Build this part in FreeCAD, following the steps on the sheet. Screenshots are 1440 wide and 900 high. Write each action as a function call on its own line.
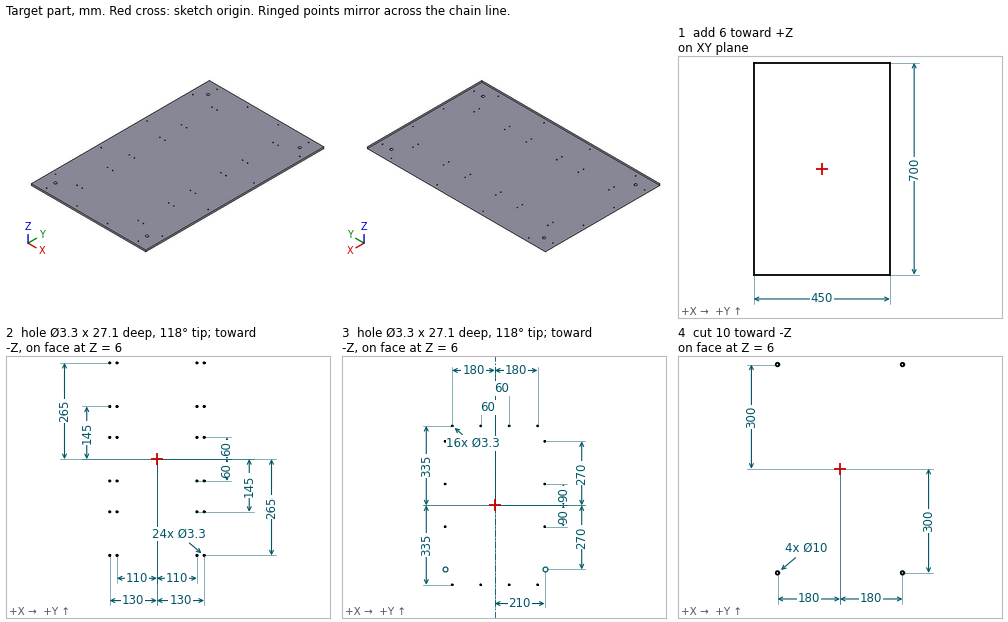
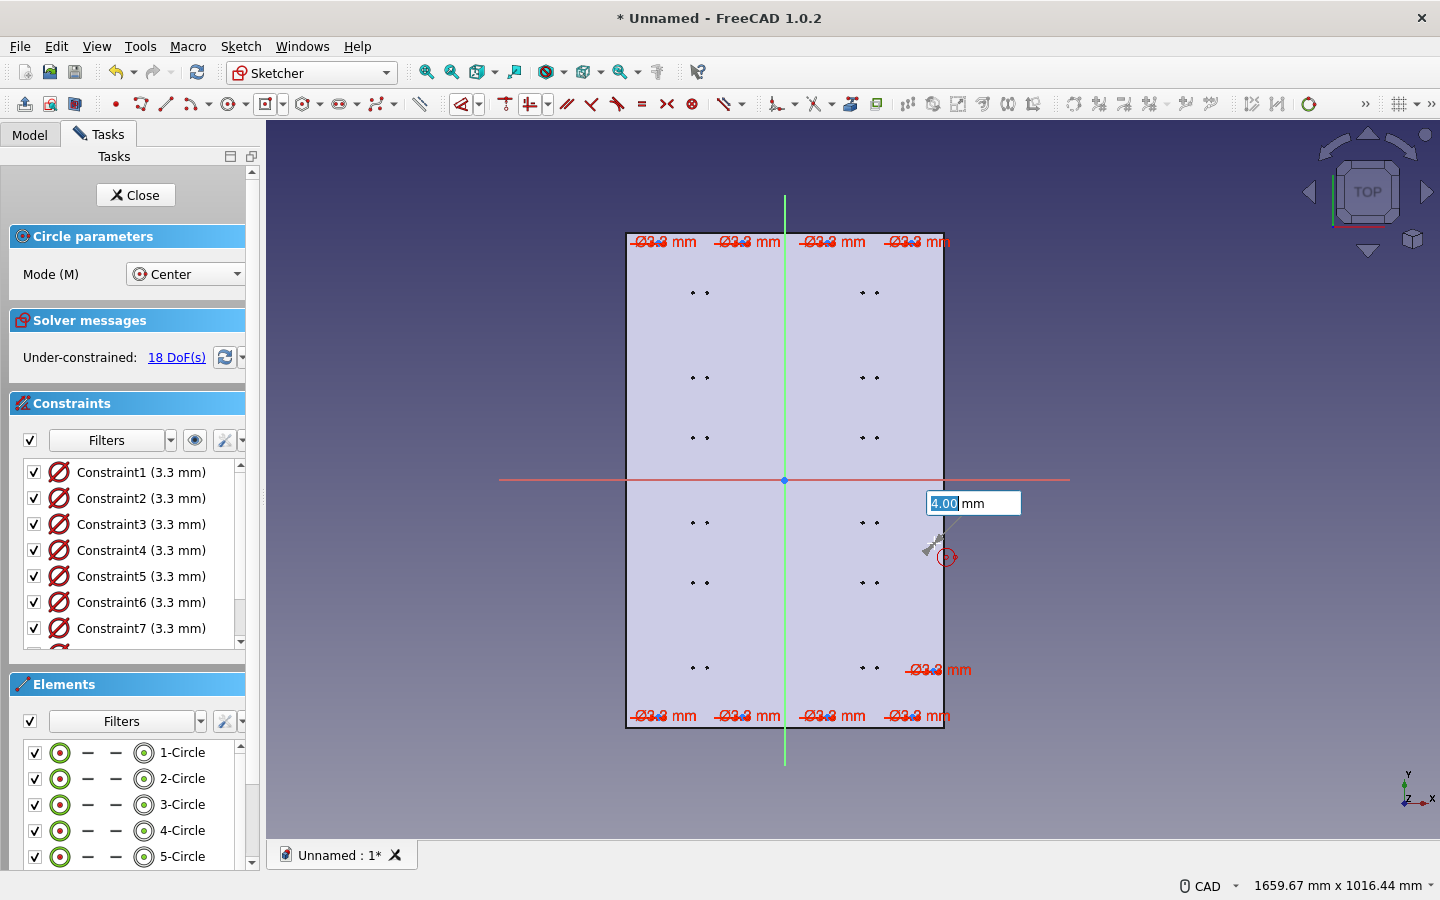
text(3.3)
key(Return)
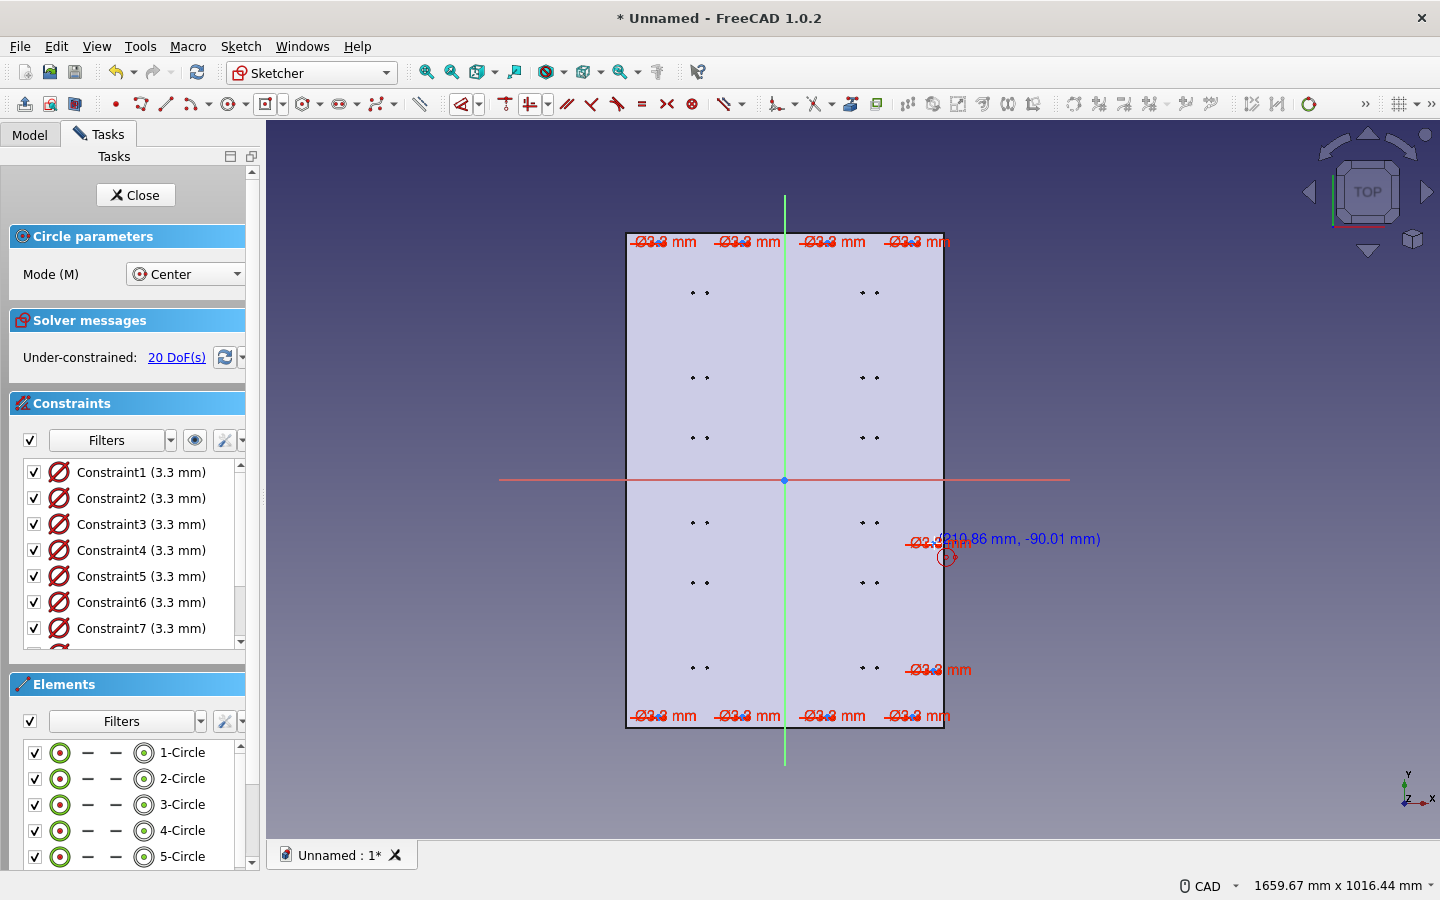
scroll(933, 417, up, 15)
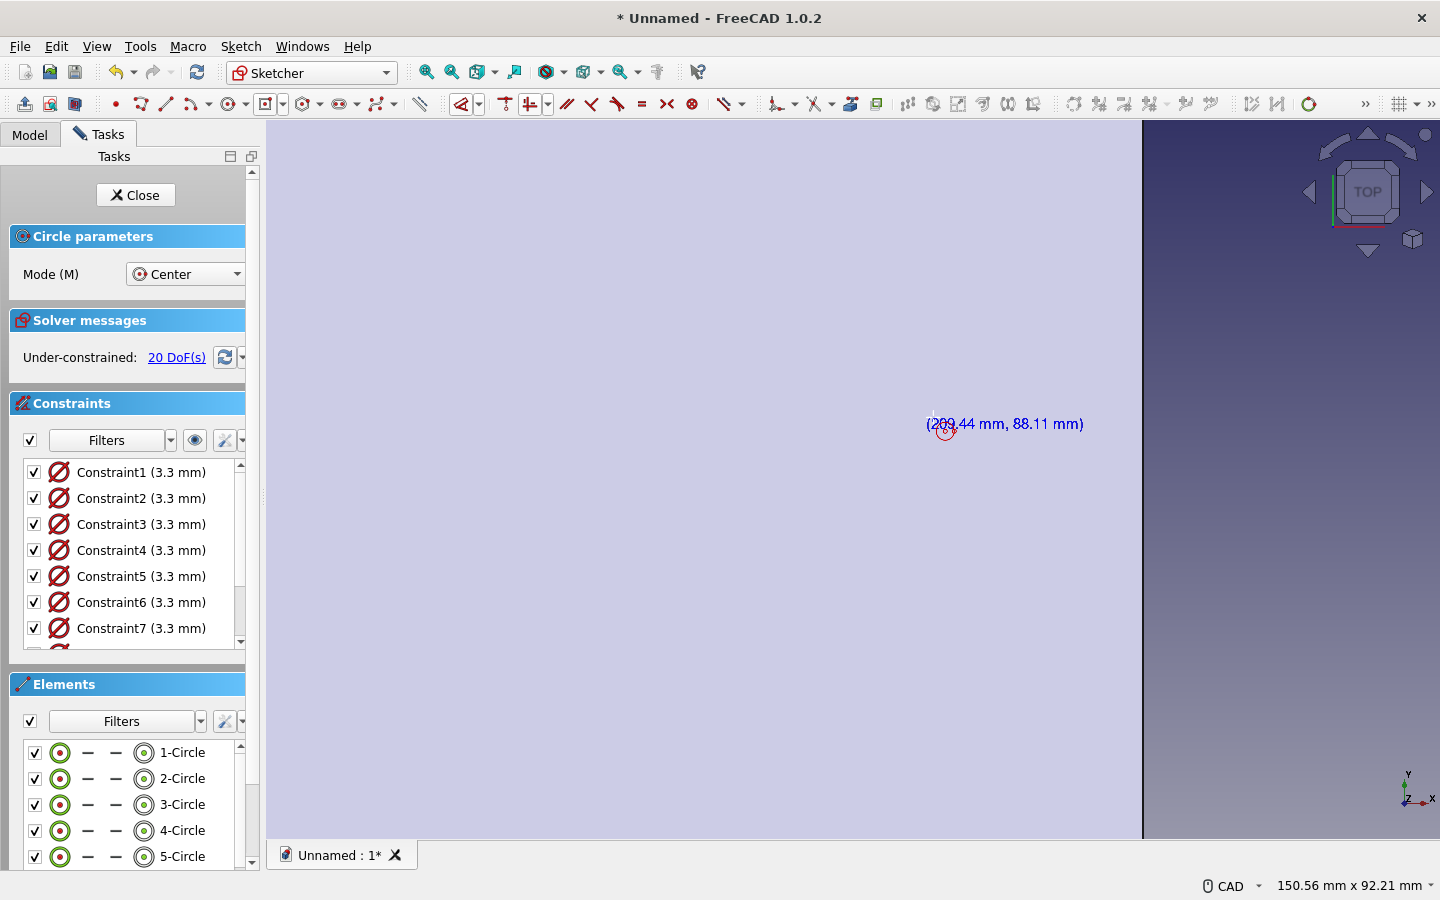
scroll(933, 417, down, 15)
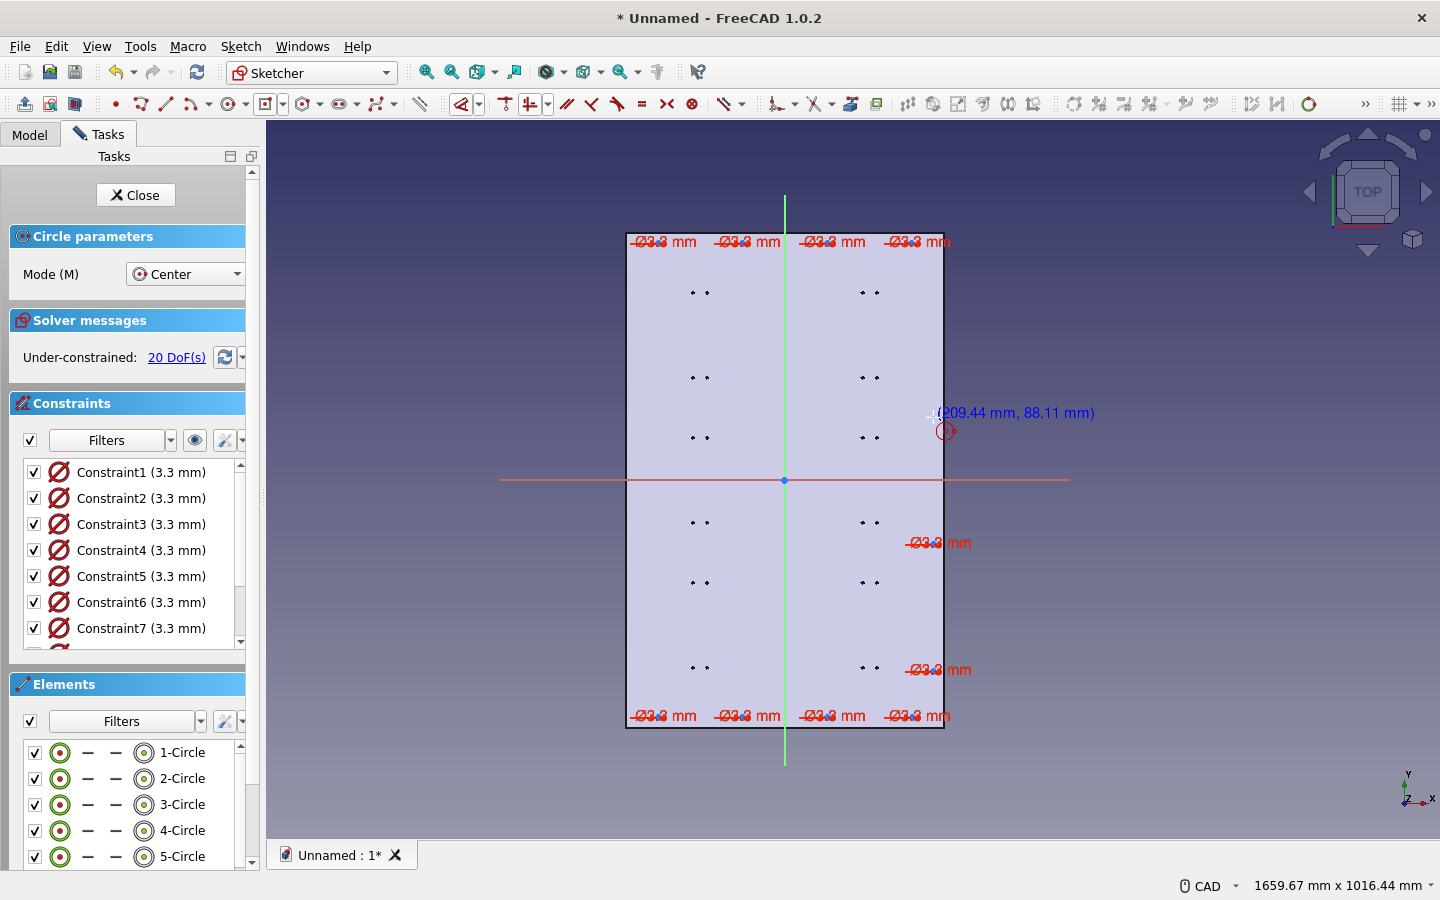
click(933, 417)
move(934, 416)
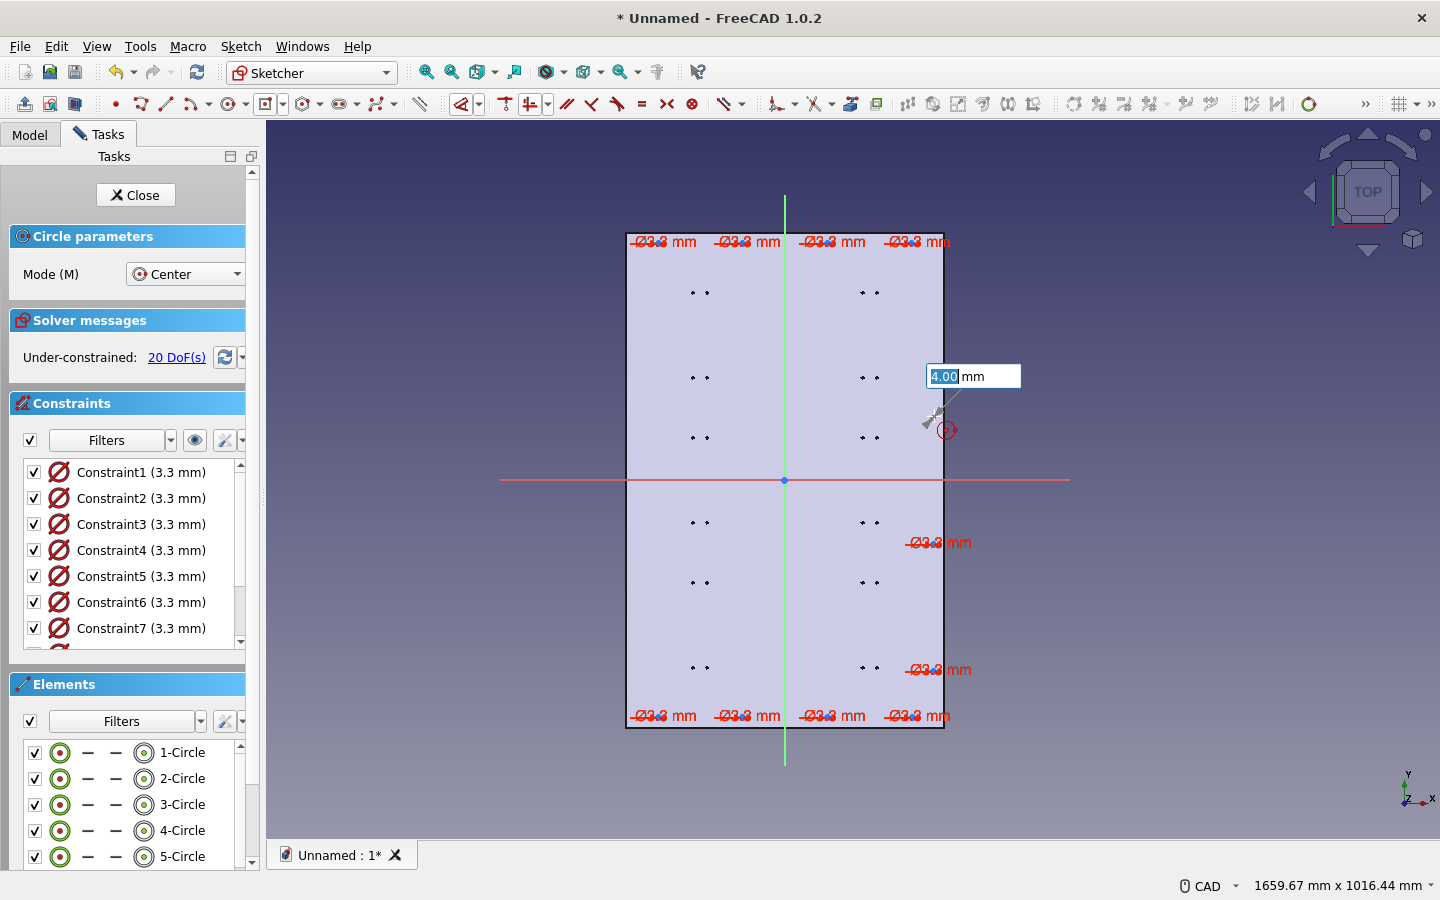
text(3.3)
key(Return)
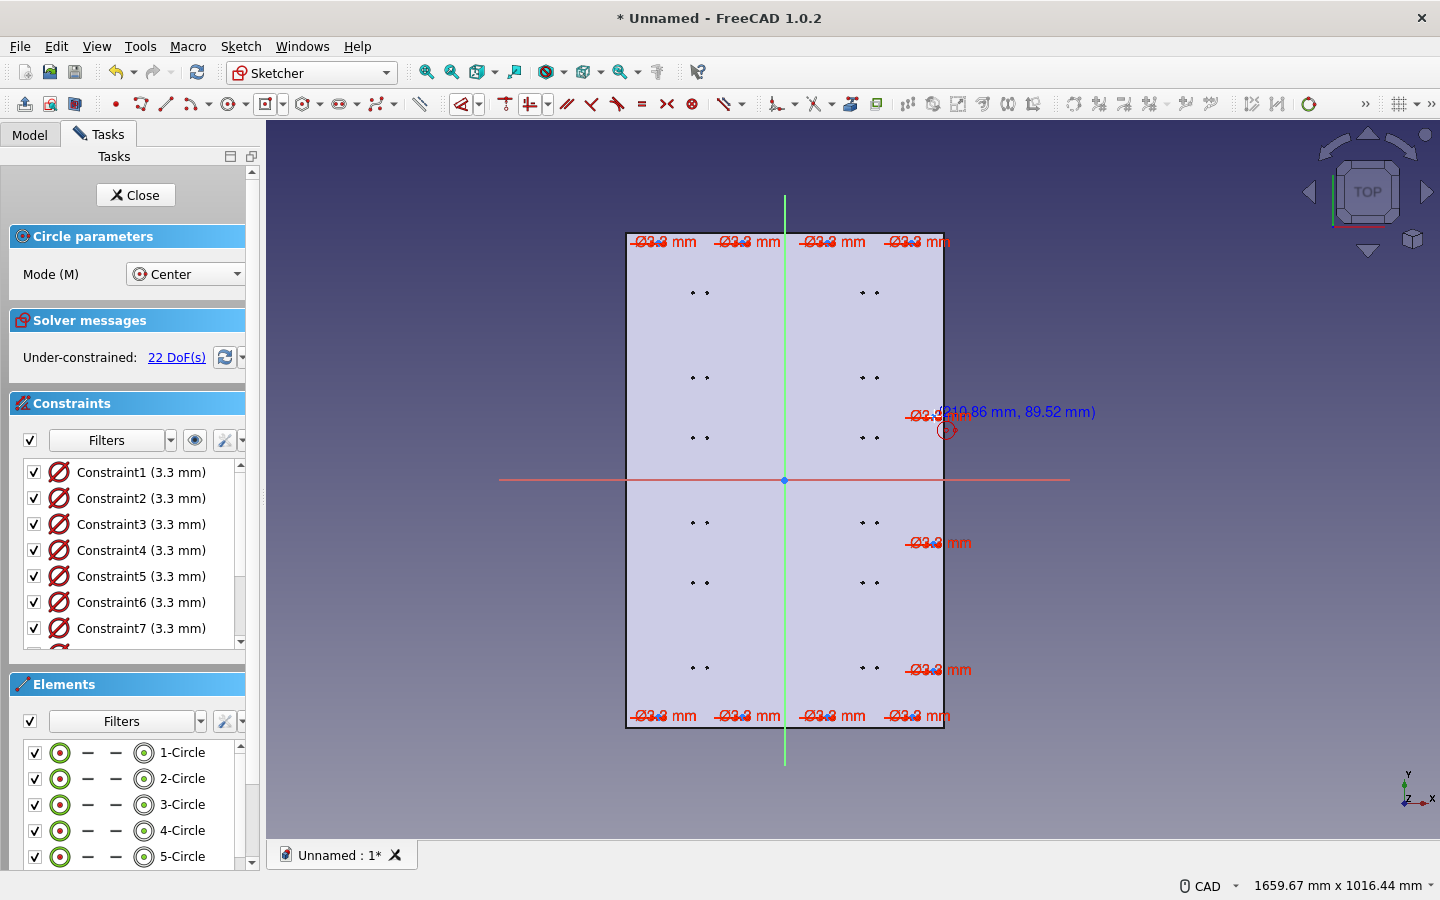
scroll(933, 289, up, 15)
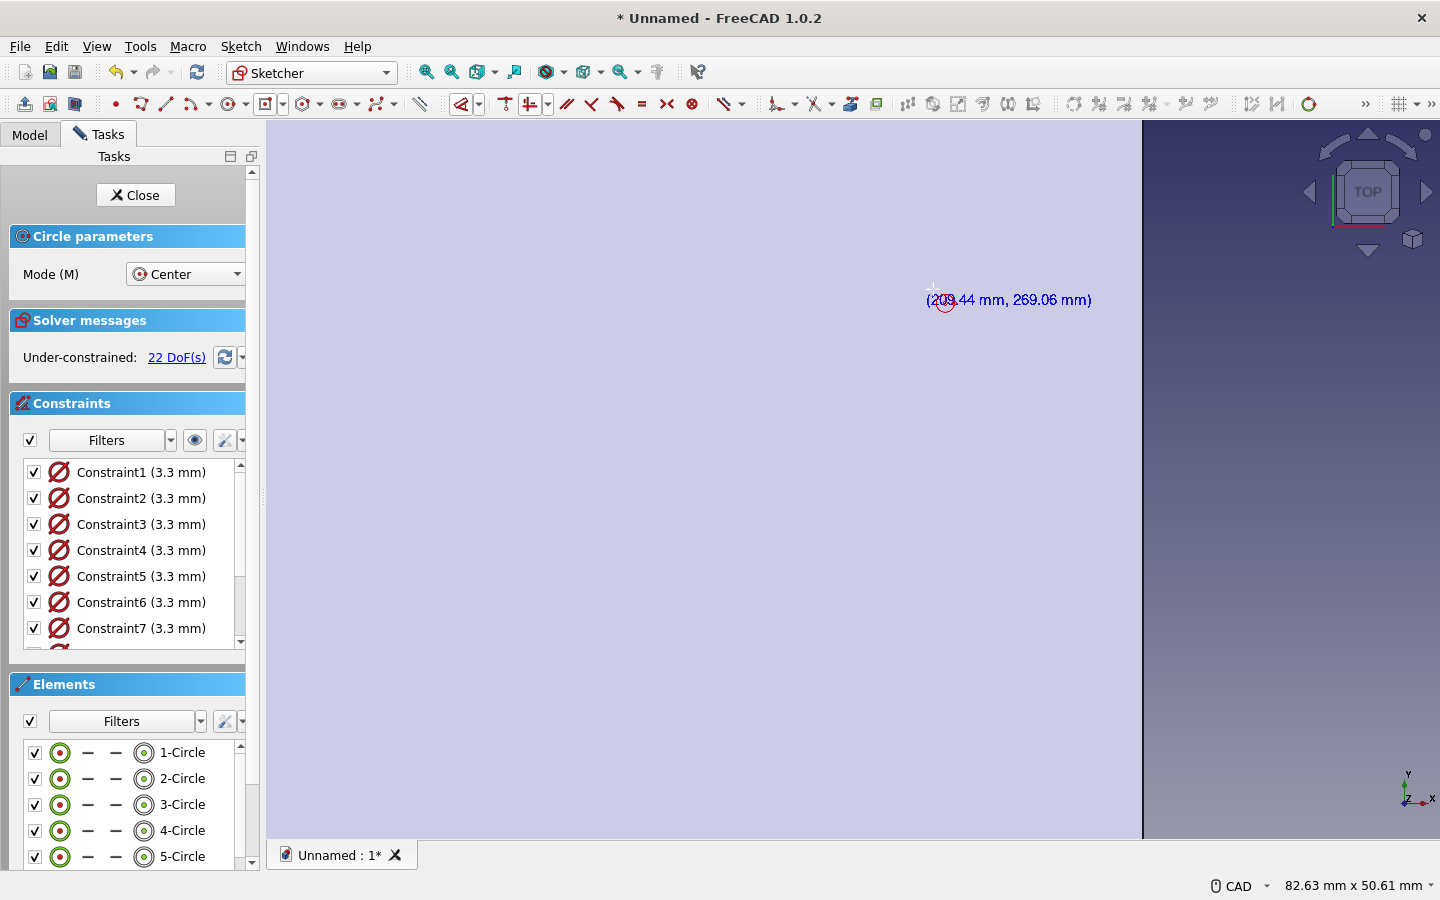
scroll(933, 288, down, 15)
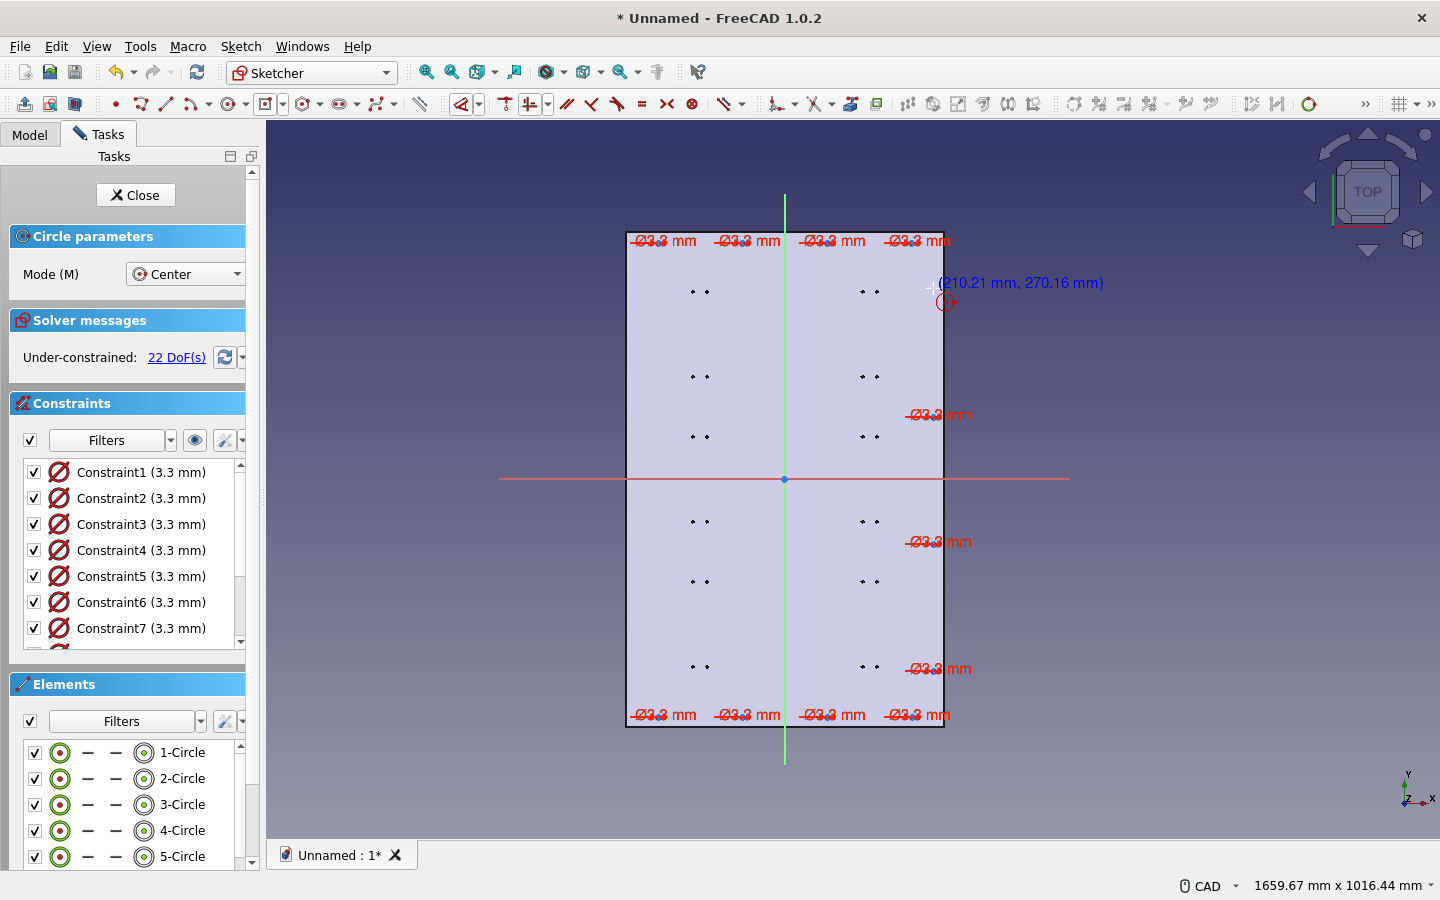
click(933, 288)
move(934, 288)